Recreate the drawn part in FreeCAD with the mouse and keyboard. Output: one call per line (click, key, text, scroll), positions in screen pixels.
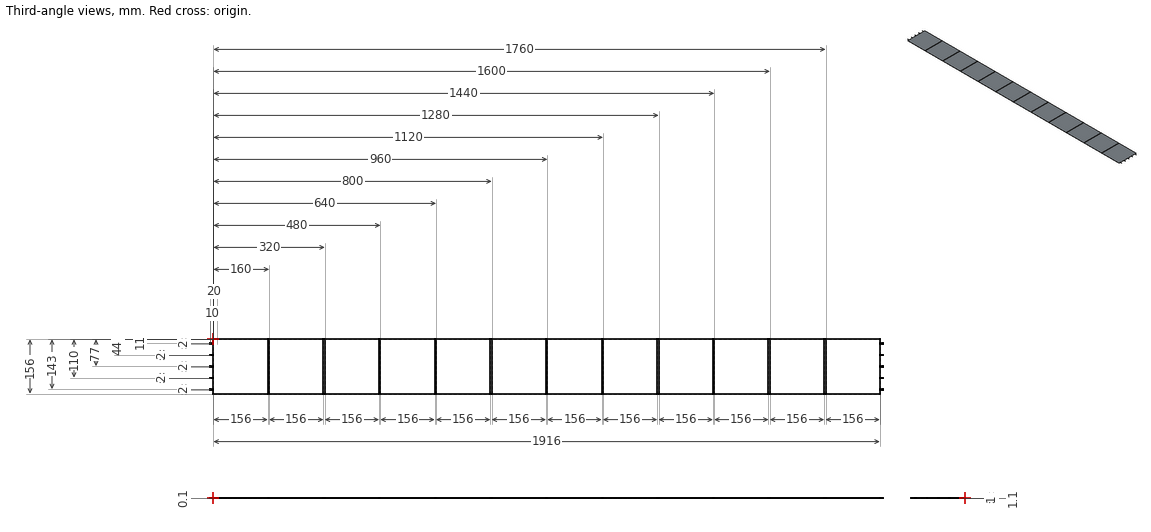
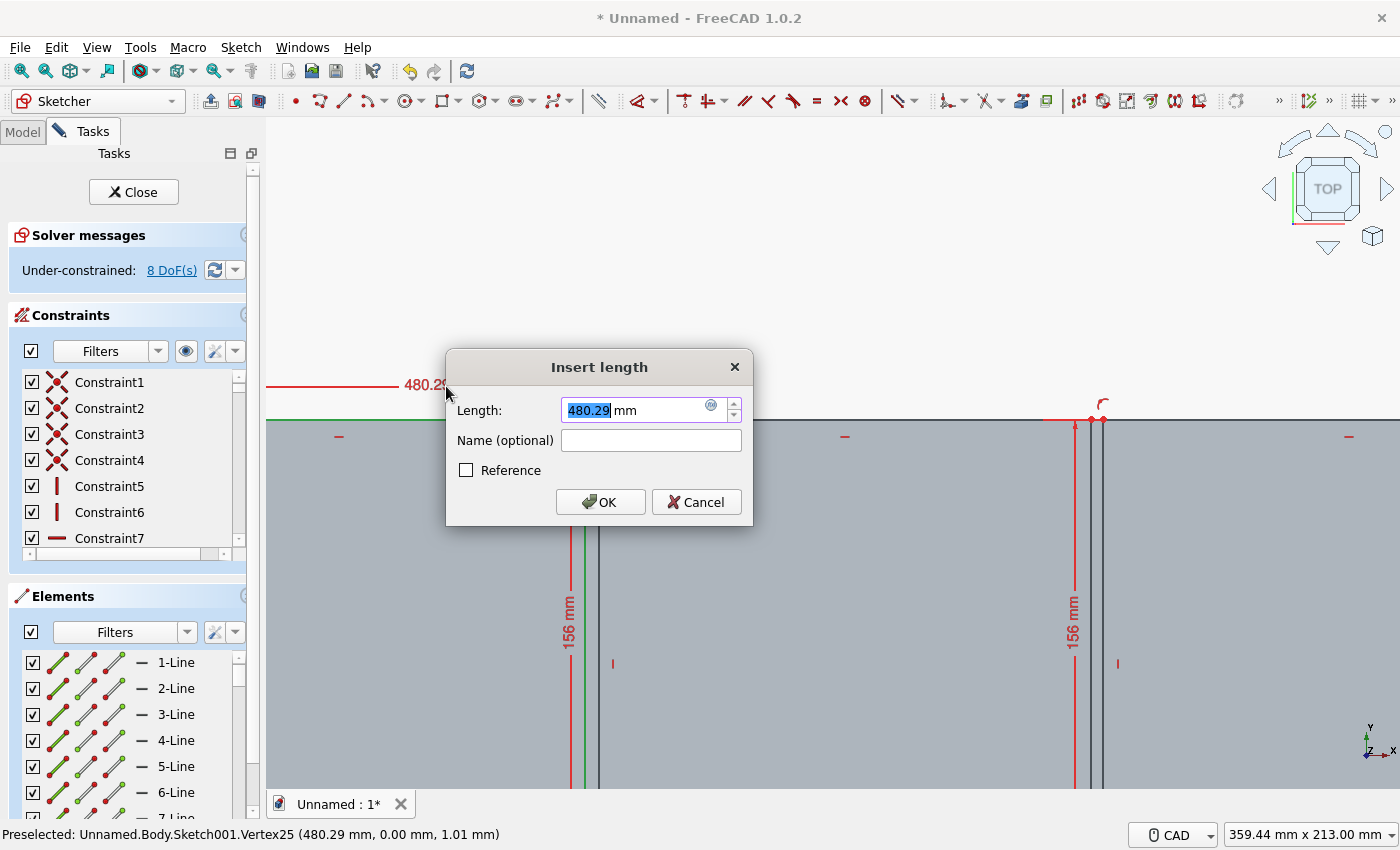
text(480)
key(Return)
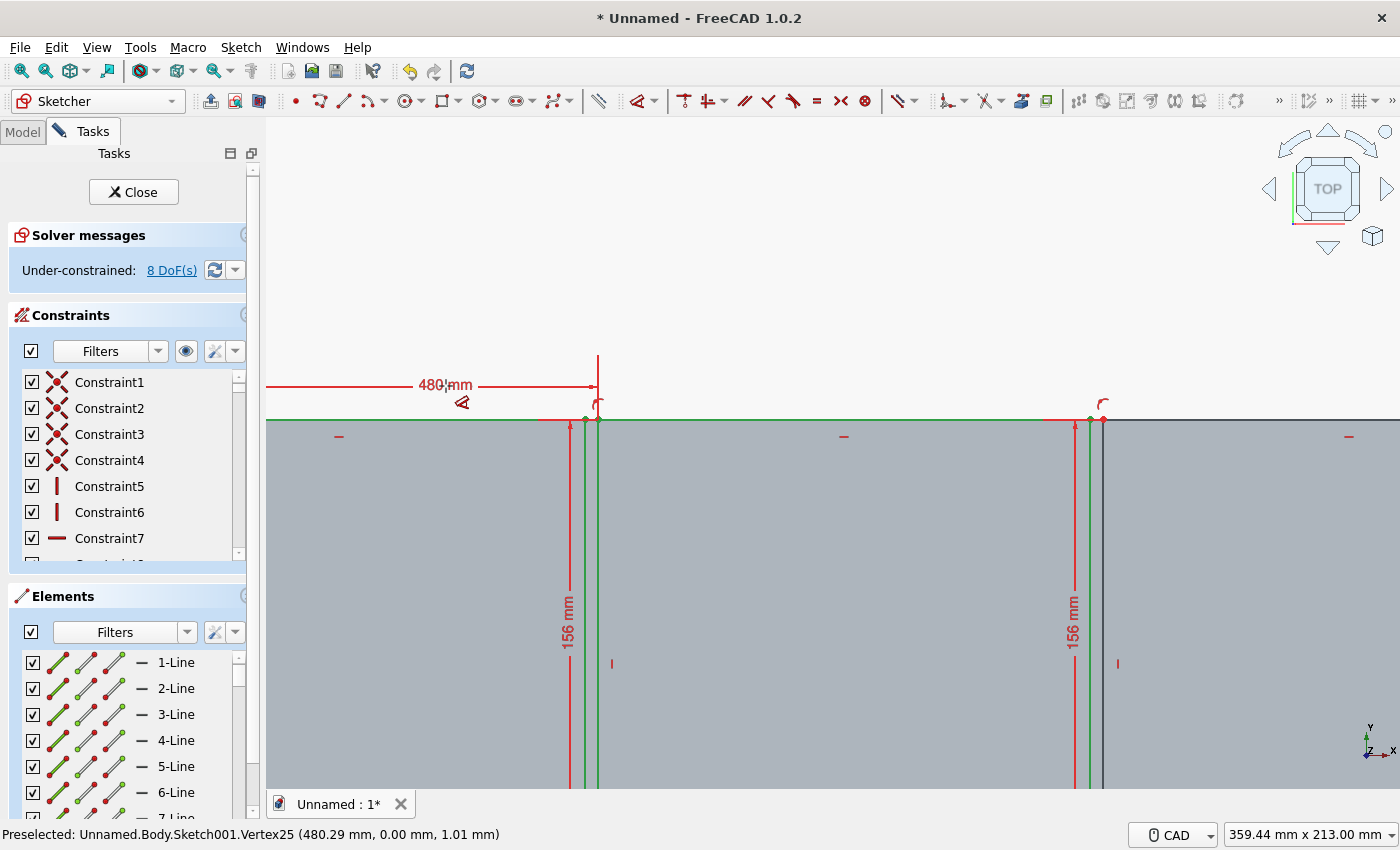
click(1103, 420)
click(699, 386)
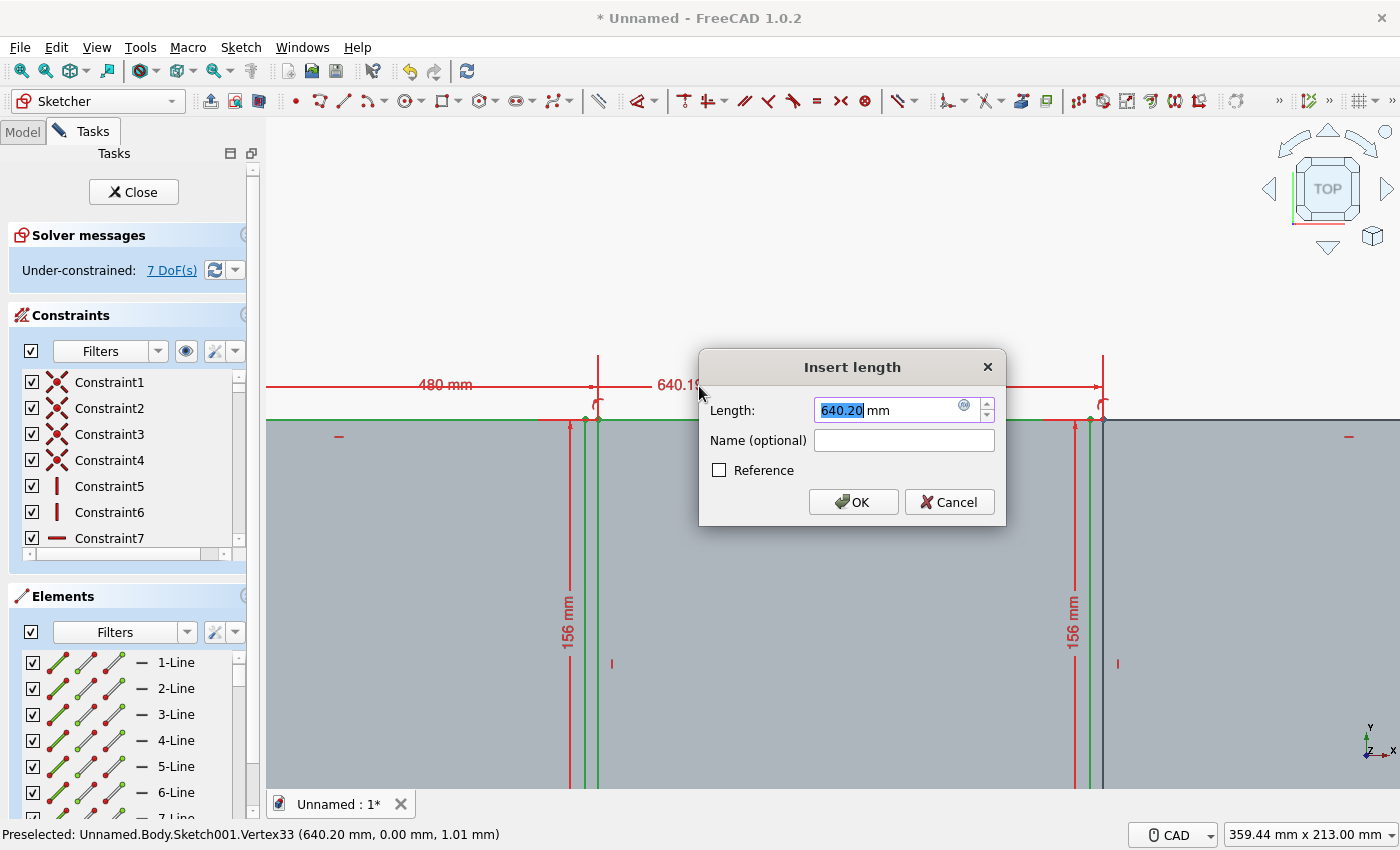
text(640)
key(Return)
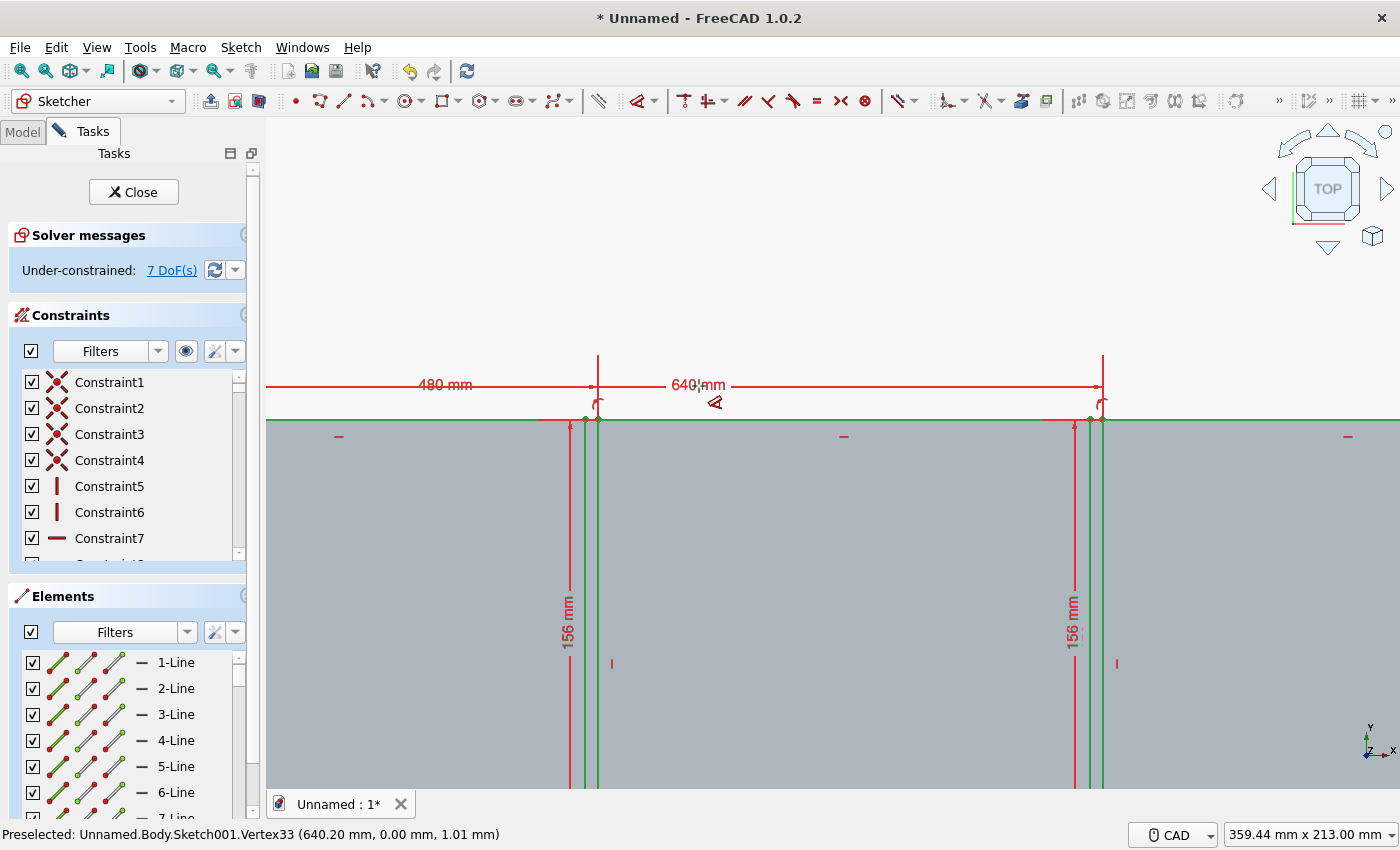
scroll(597, 426, down, 11)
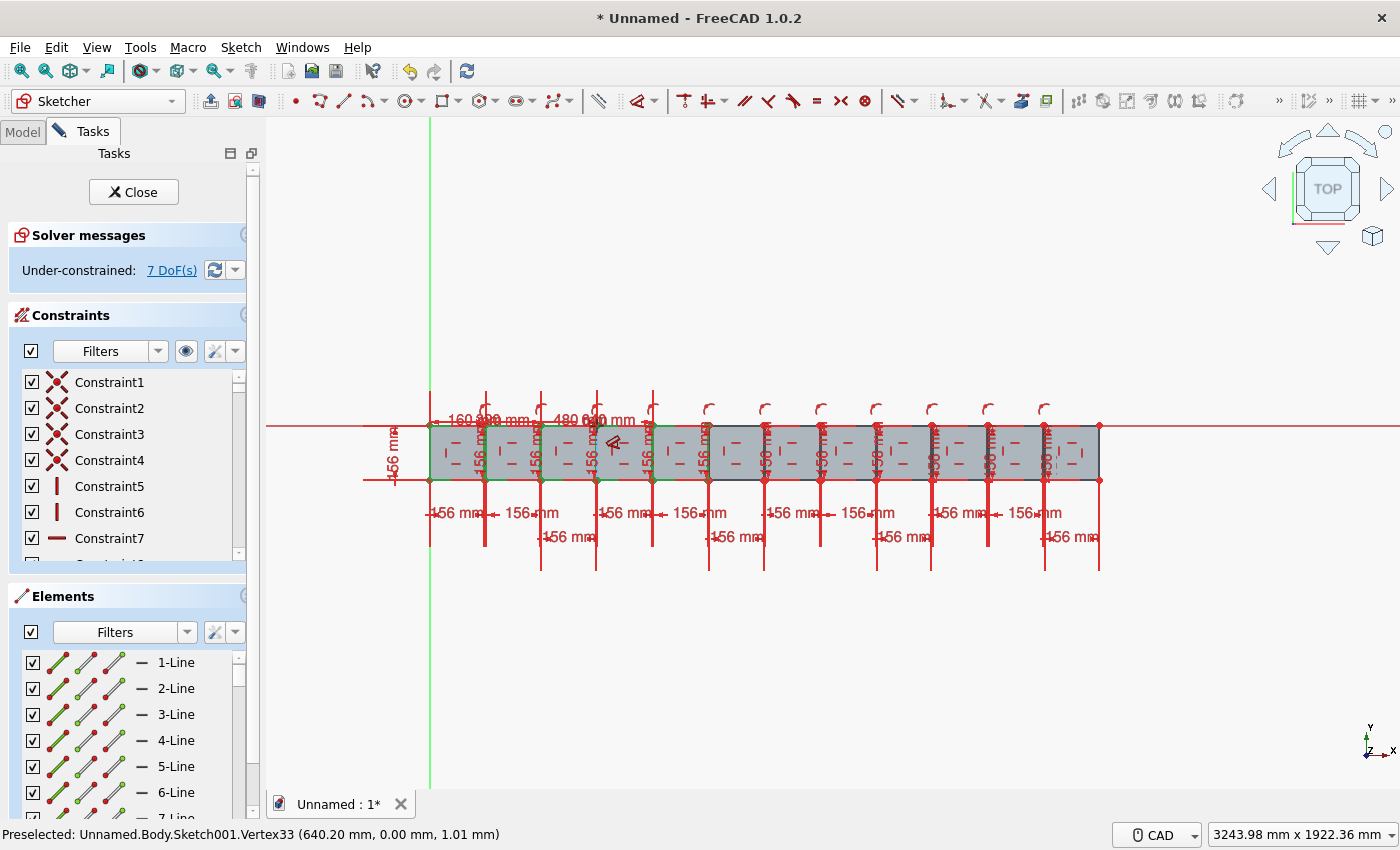
scroll(709, 426, up, 11)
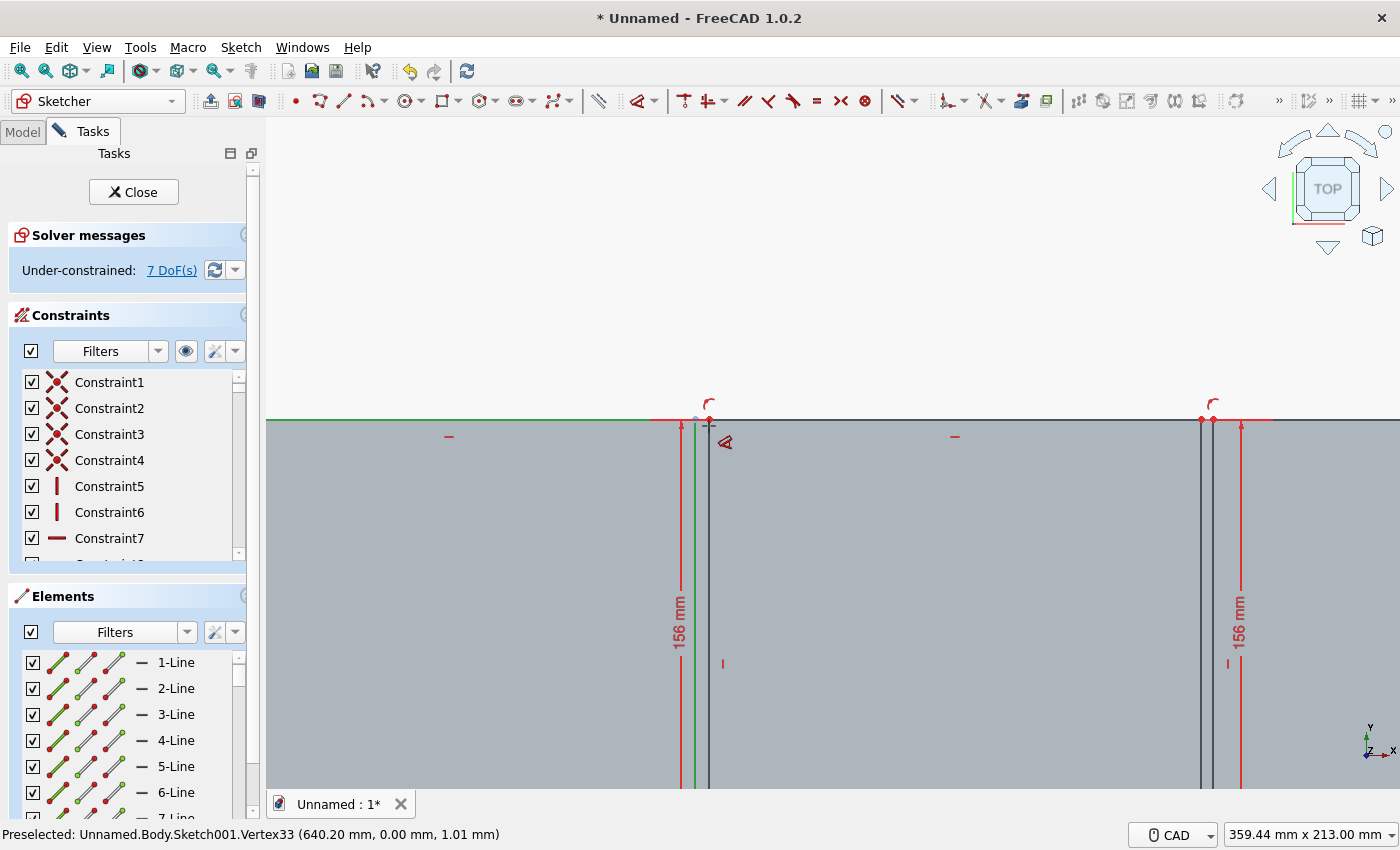
click(709, 420)
click(502, 386)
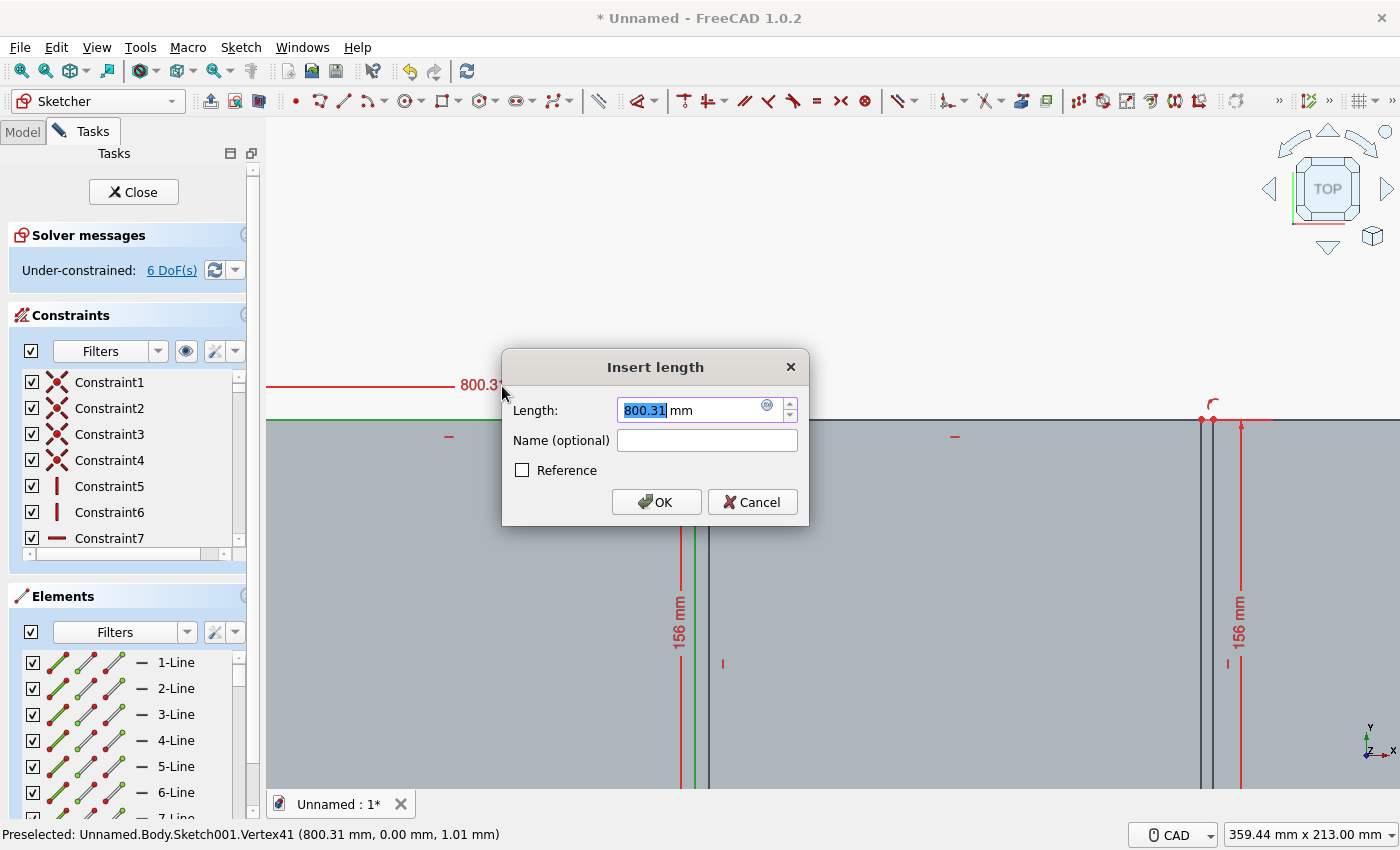
text(800)
key(Return)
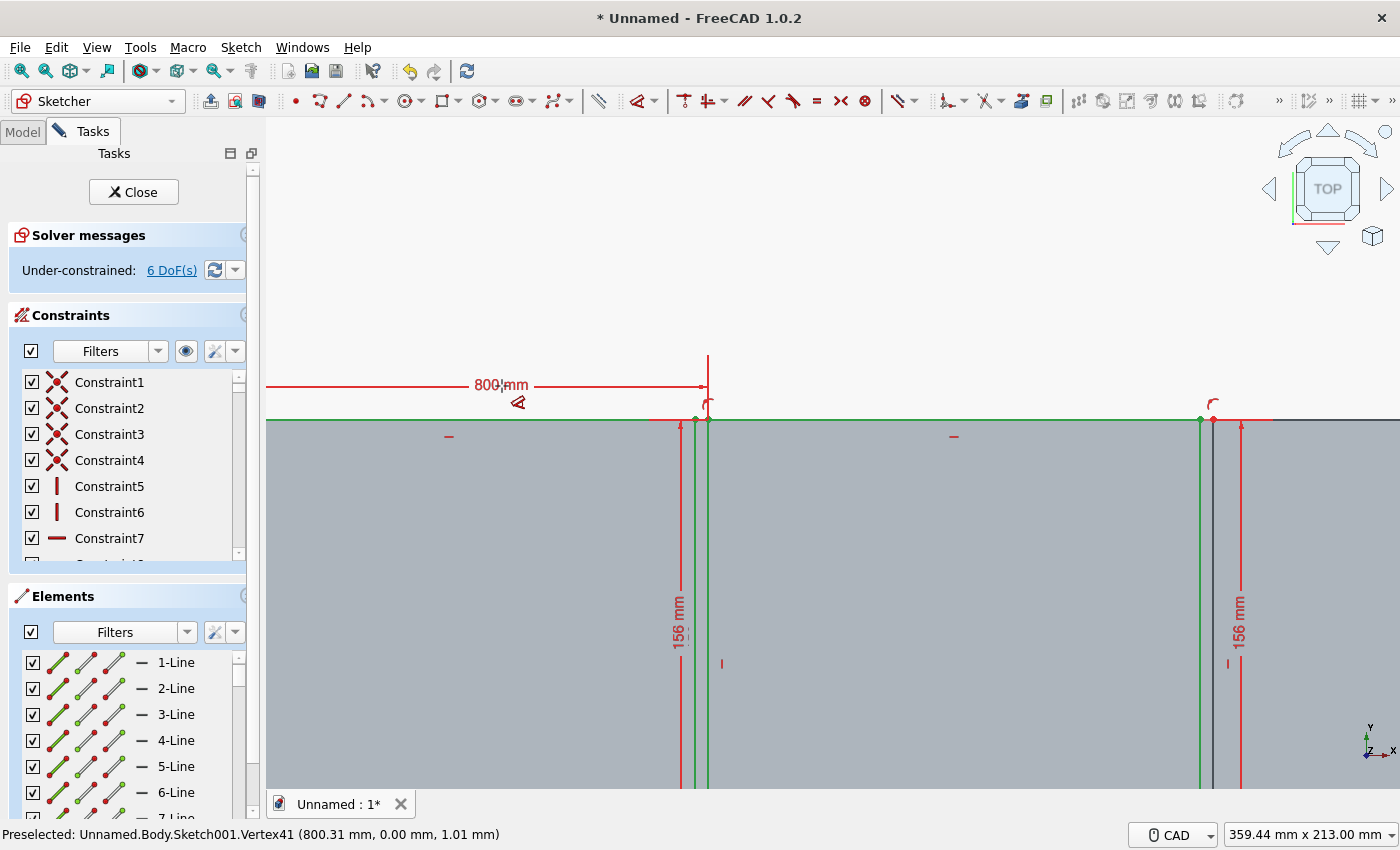
click(1213, 420)
click(754, 386)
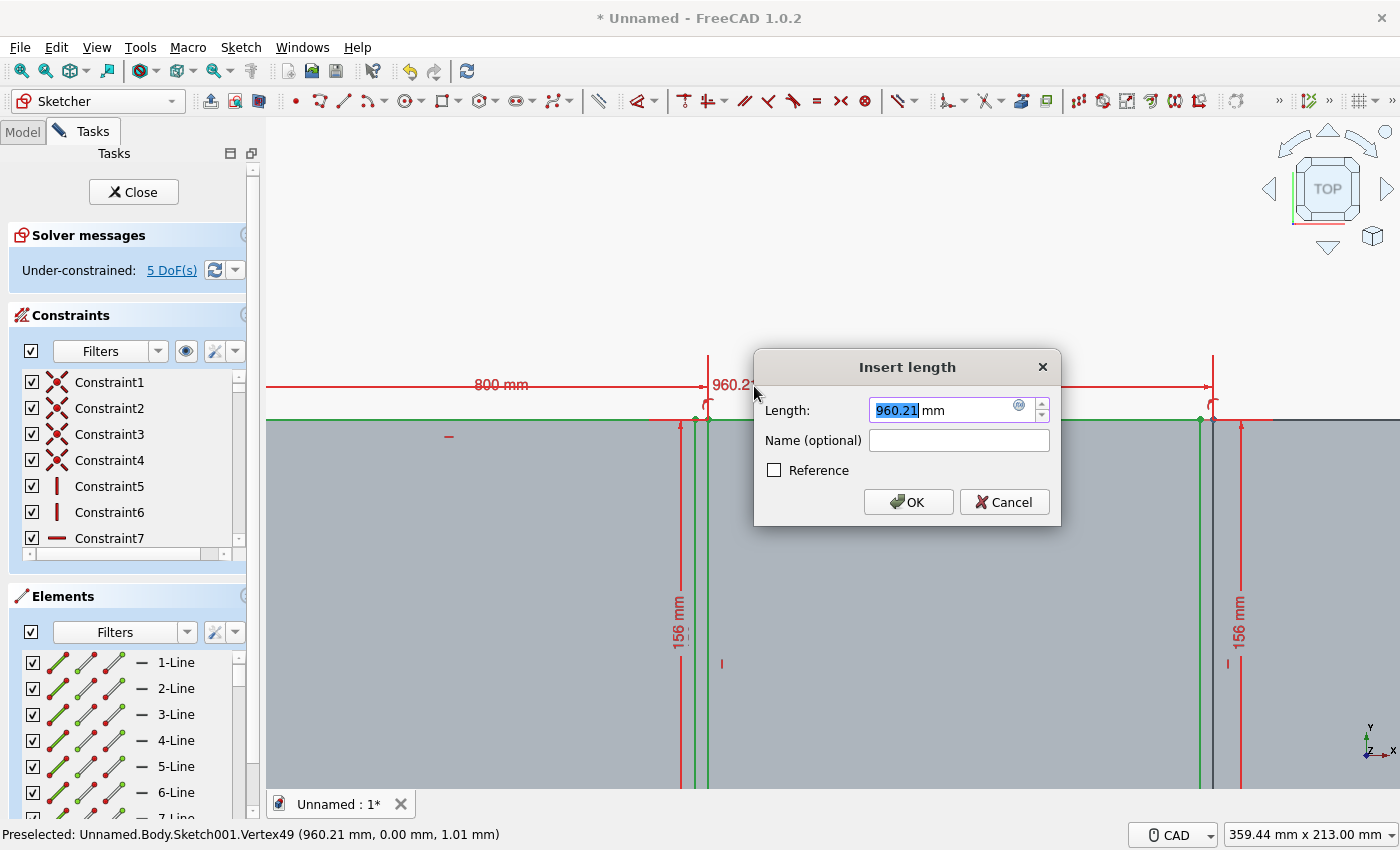
text(960)
key(Return)